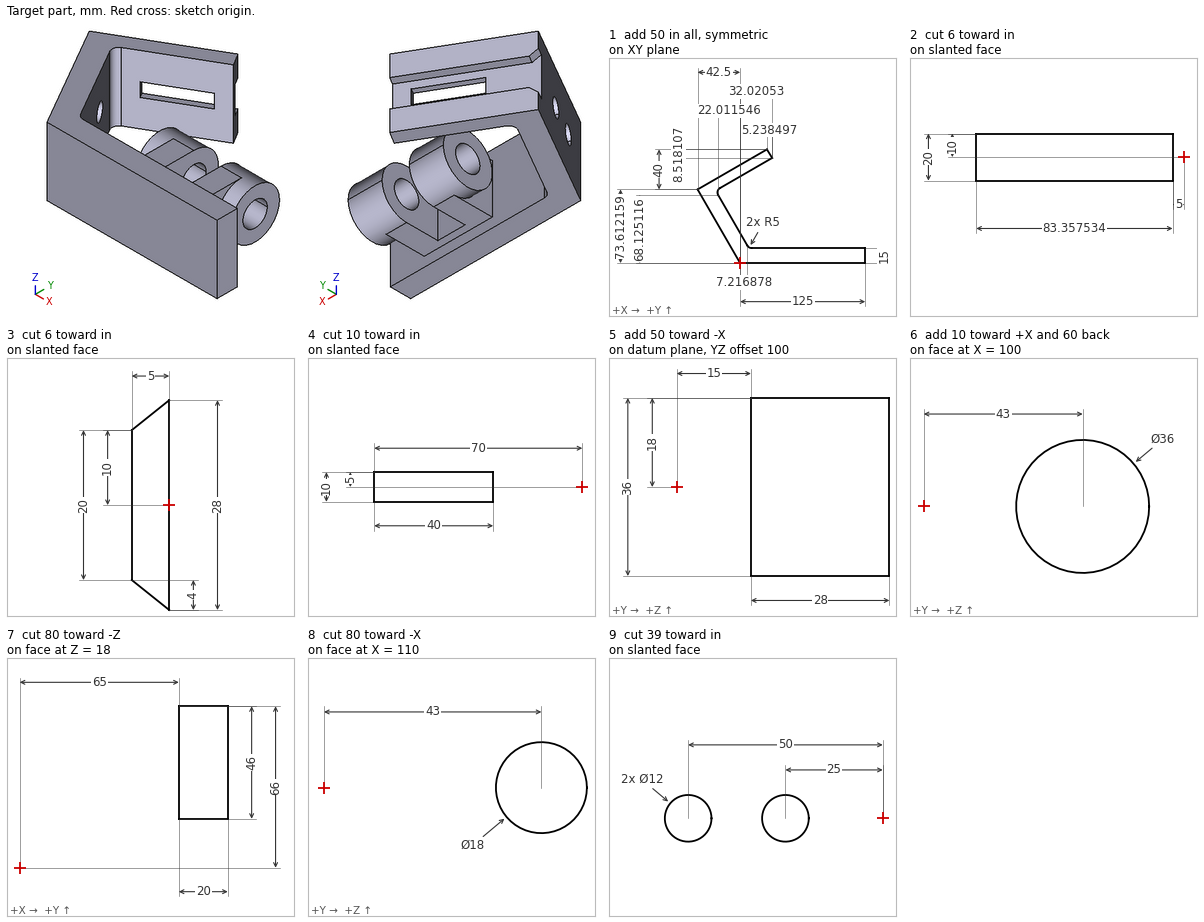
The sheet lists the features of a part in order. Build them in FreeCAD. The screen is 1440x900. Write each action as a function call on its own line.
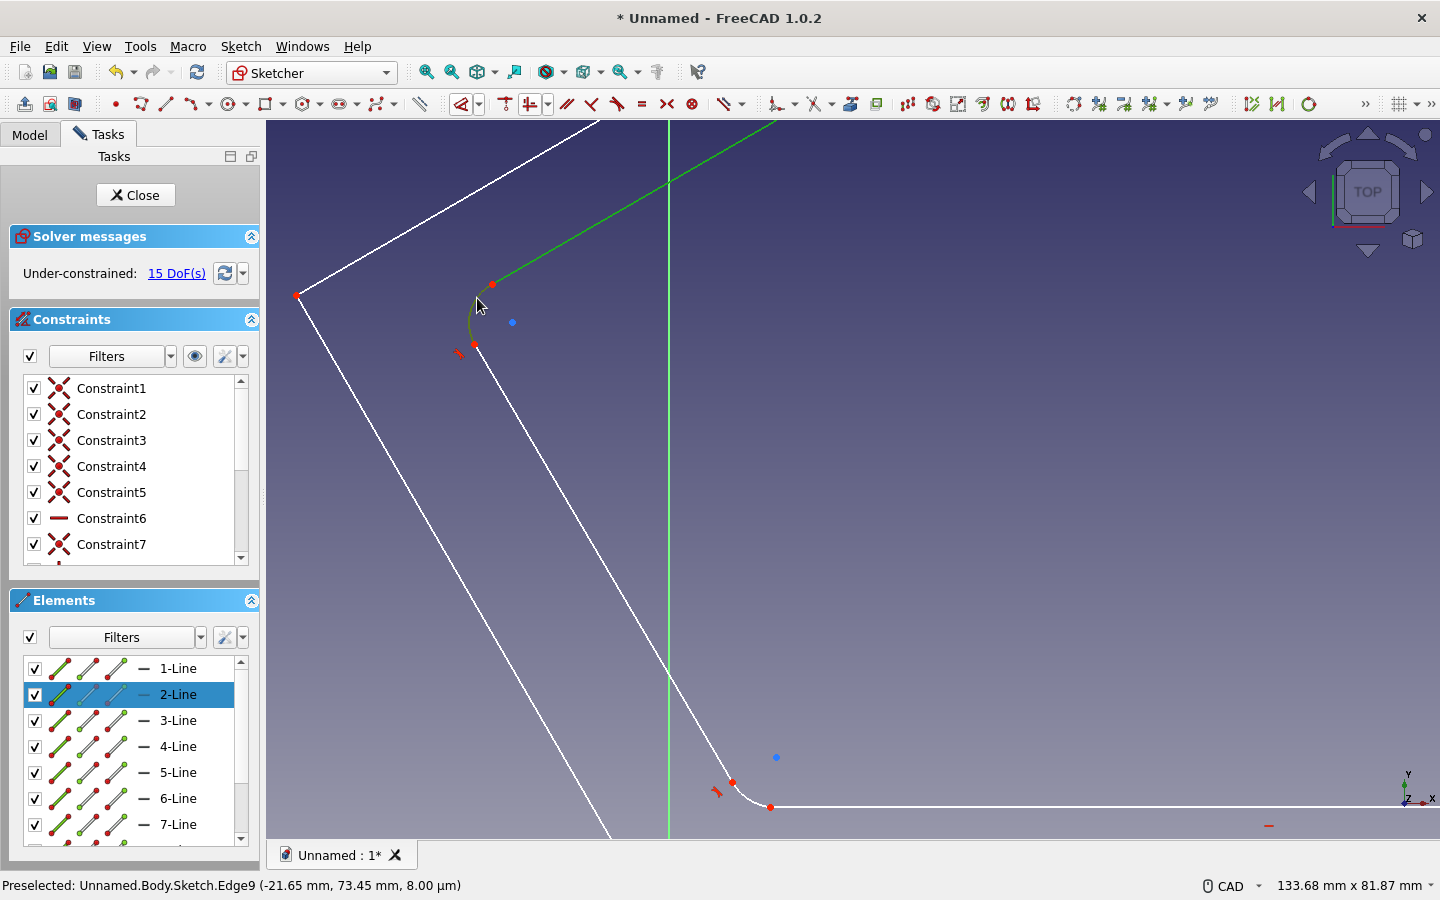
key(t)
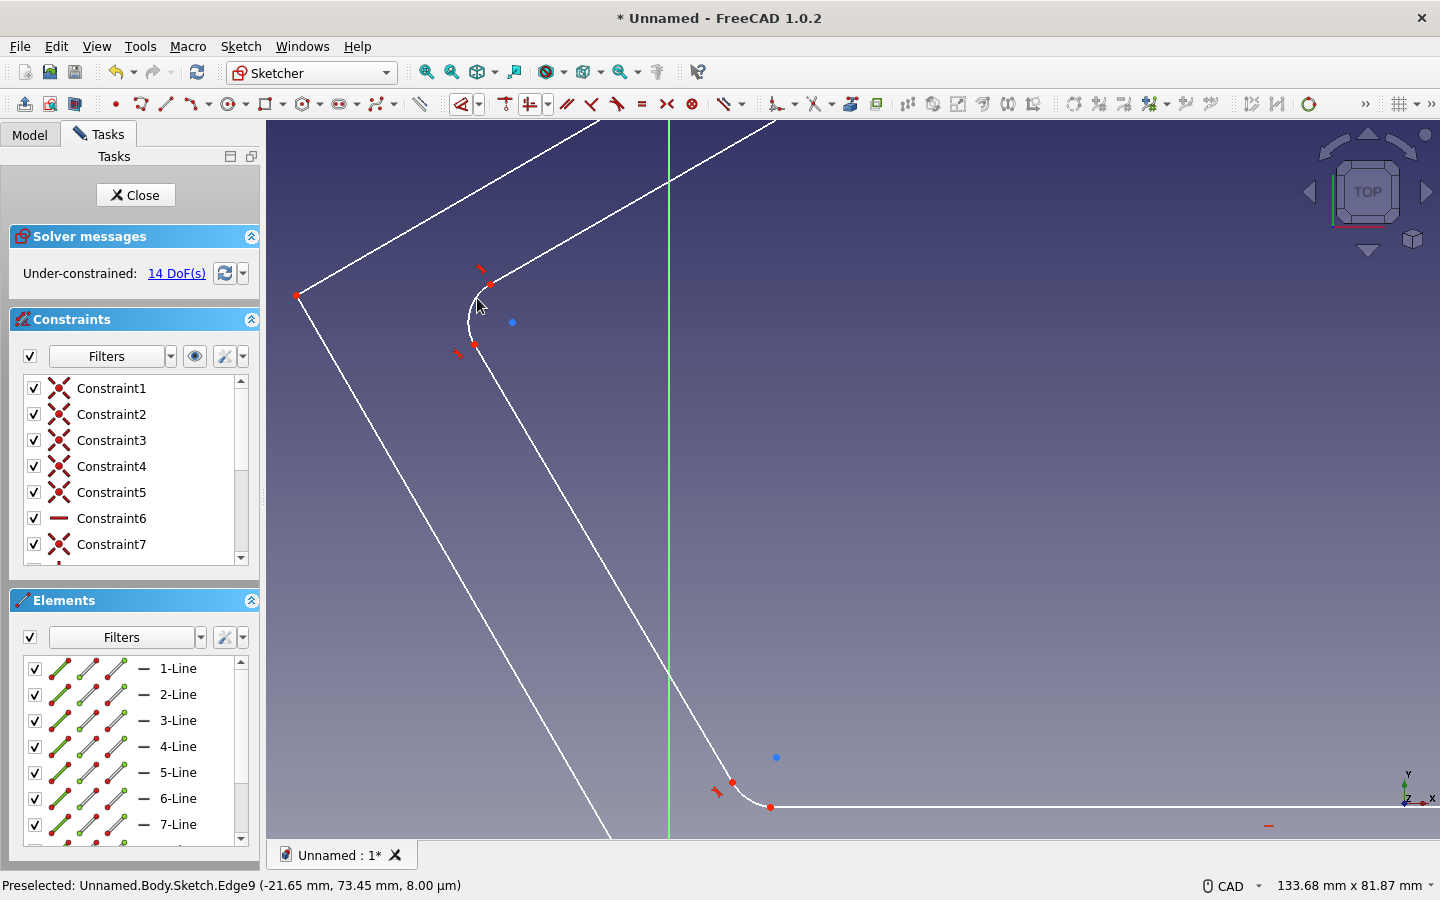
click(1070, 807)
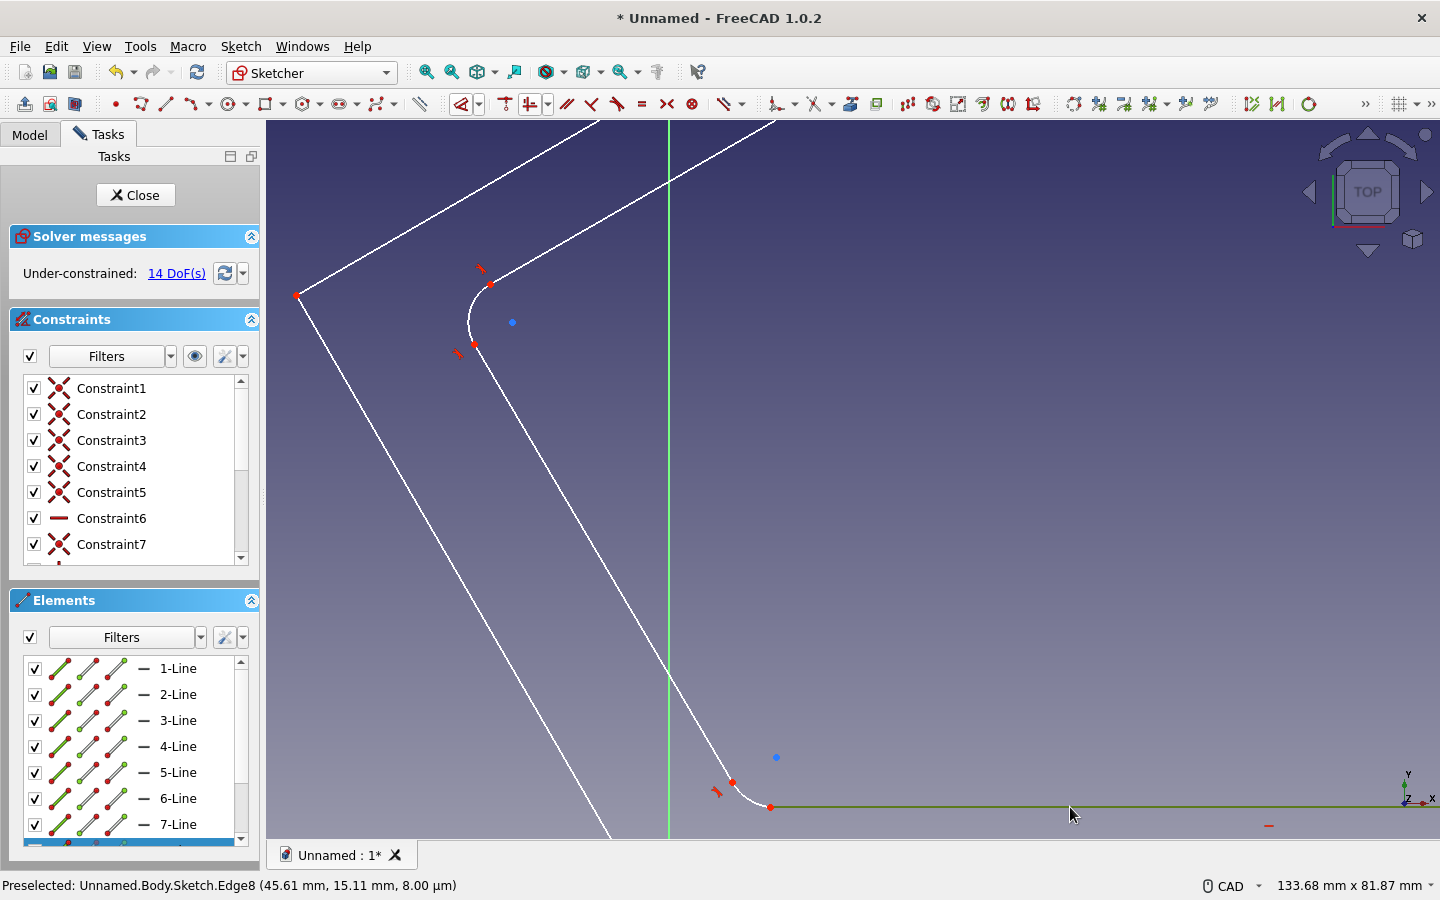
click(741, 794)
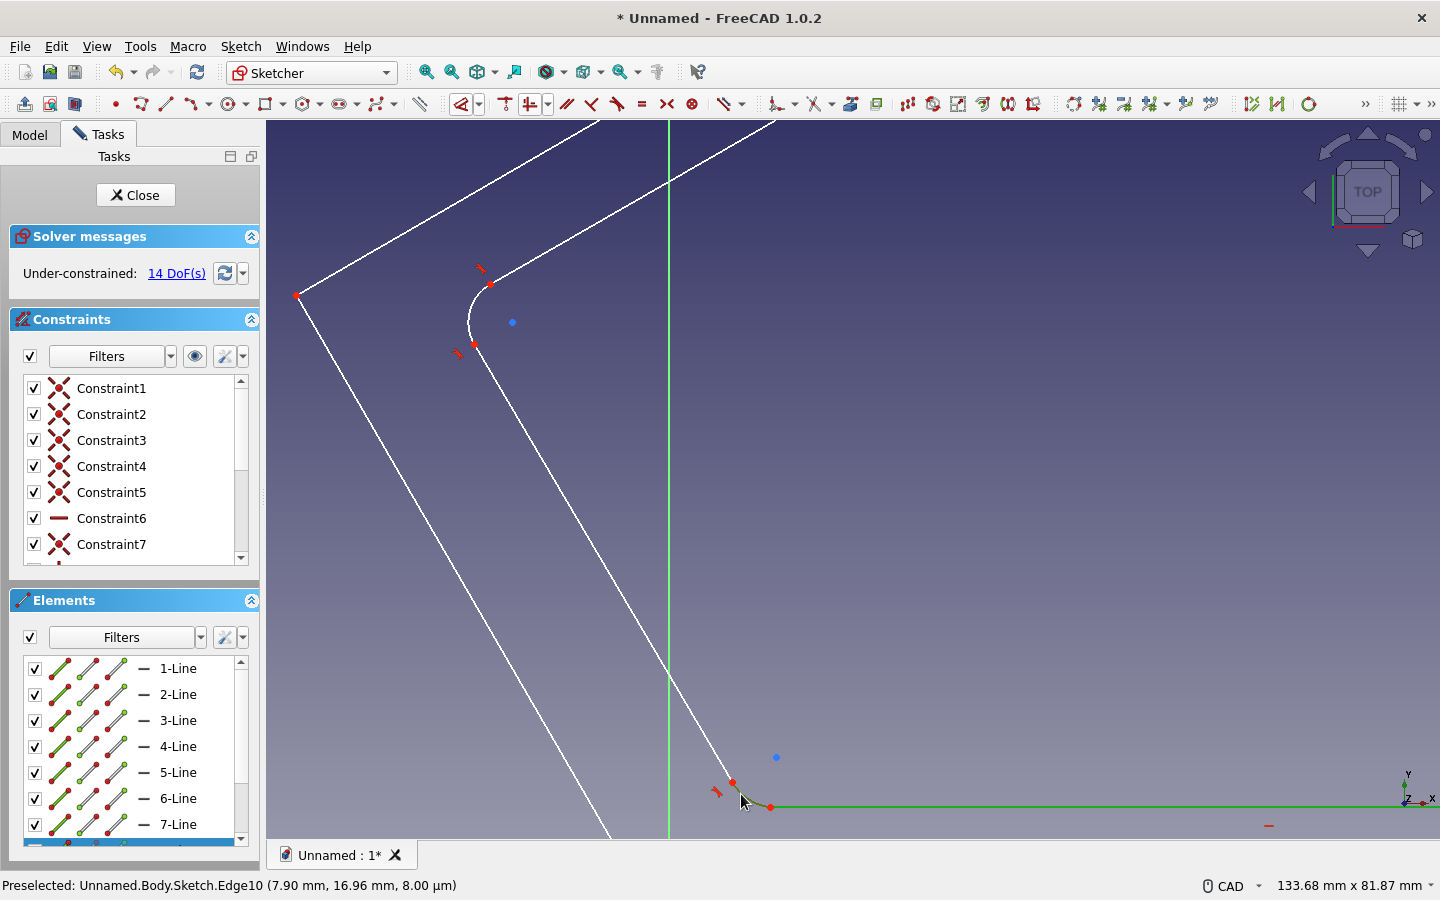
key(t)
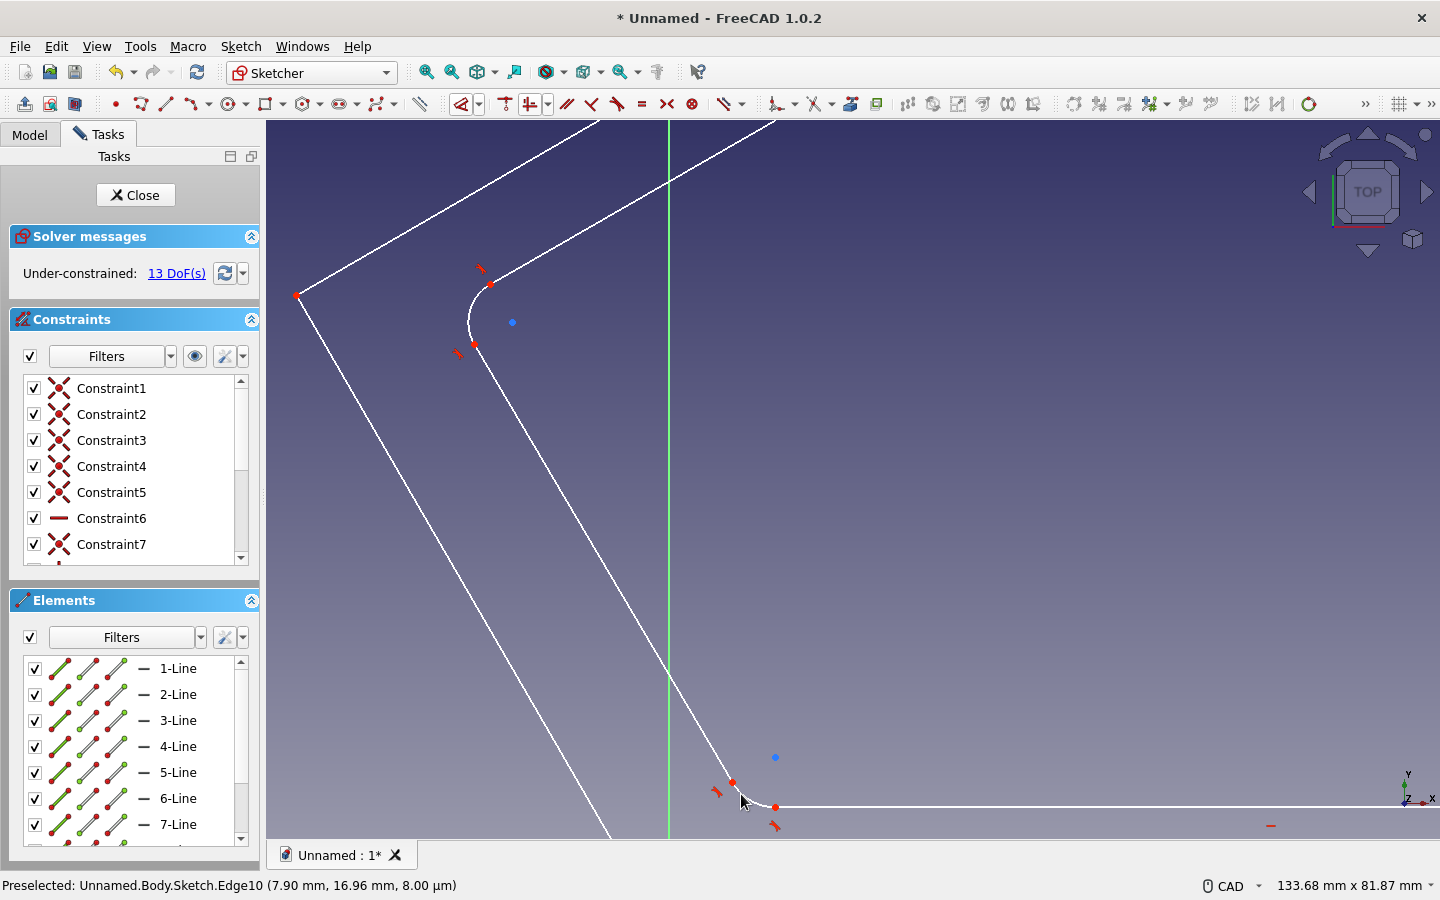
click(475, 299)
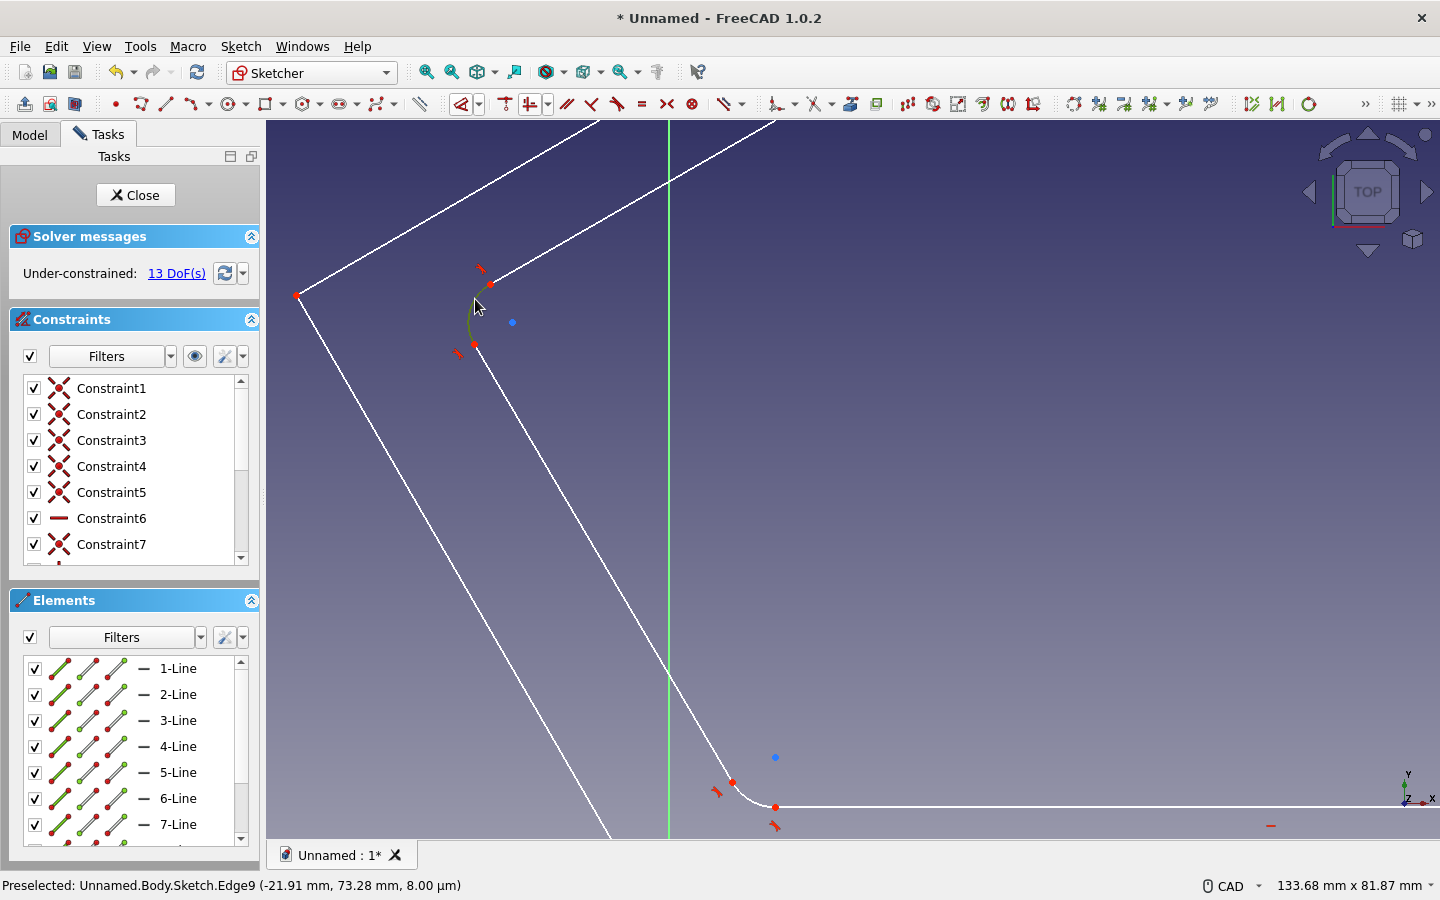
click(743, 795)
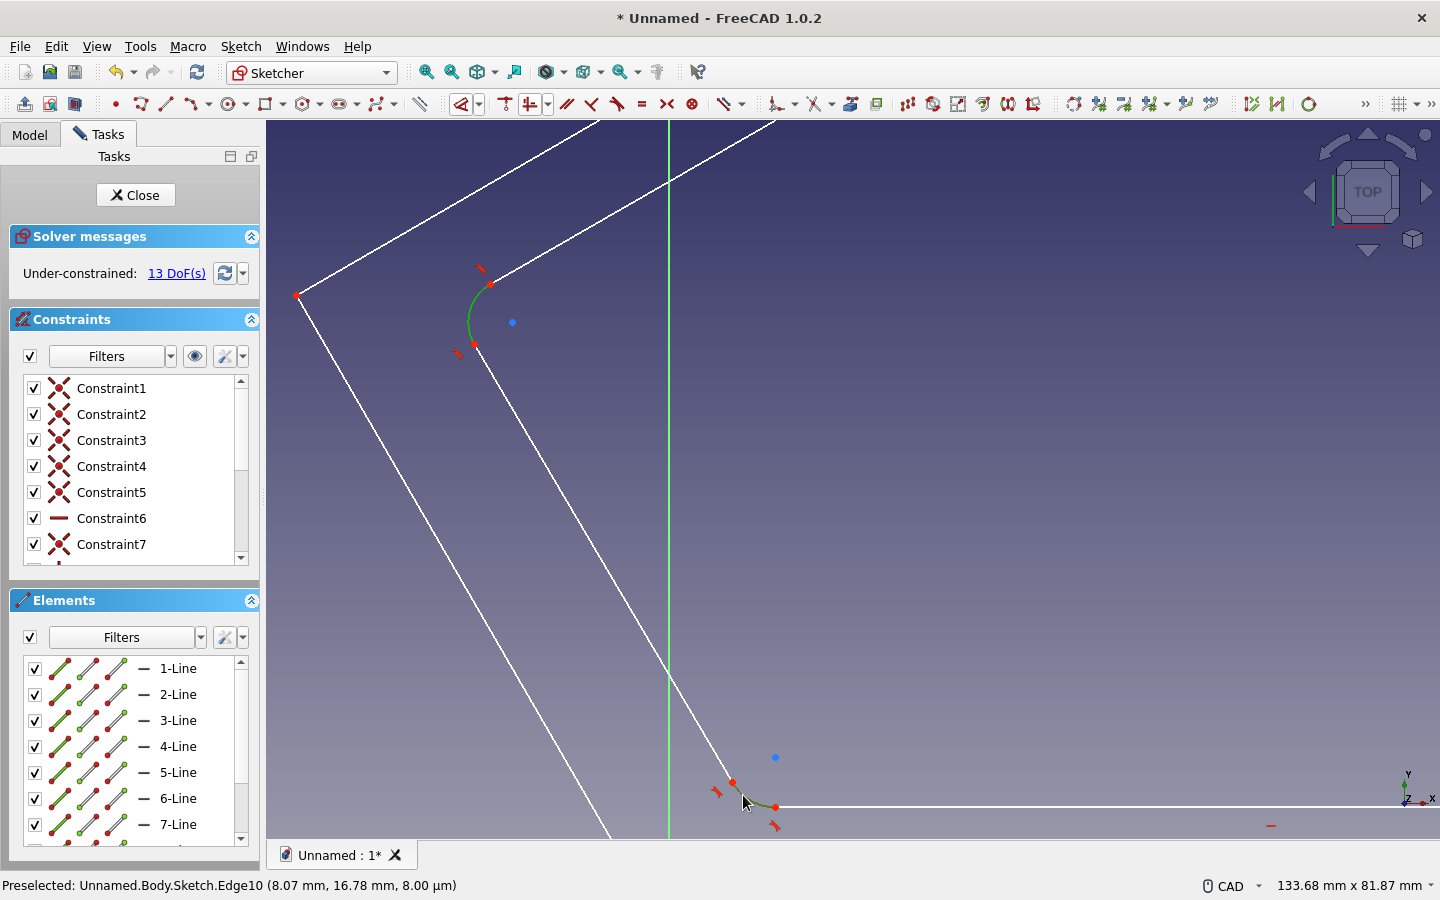
click(642, 104)